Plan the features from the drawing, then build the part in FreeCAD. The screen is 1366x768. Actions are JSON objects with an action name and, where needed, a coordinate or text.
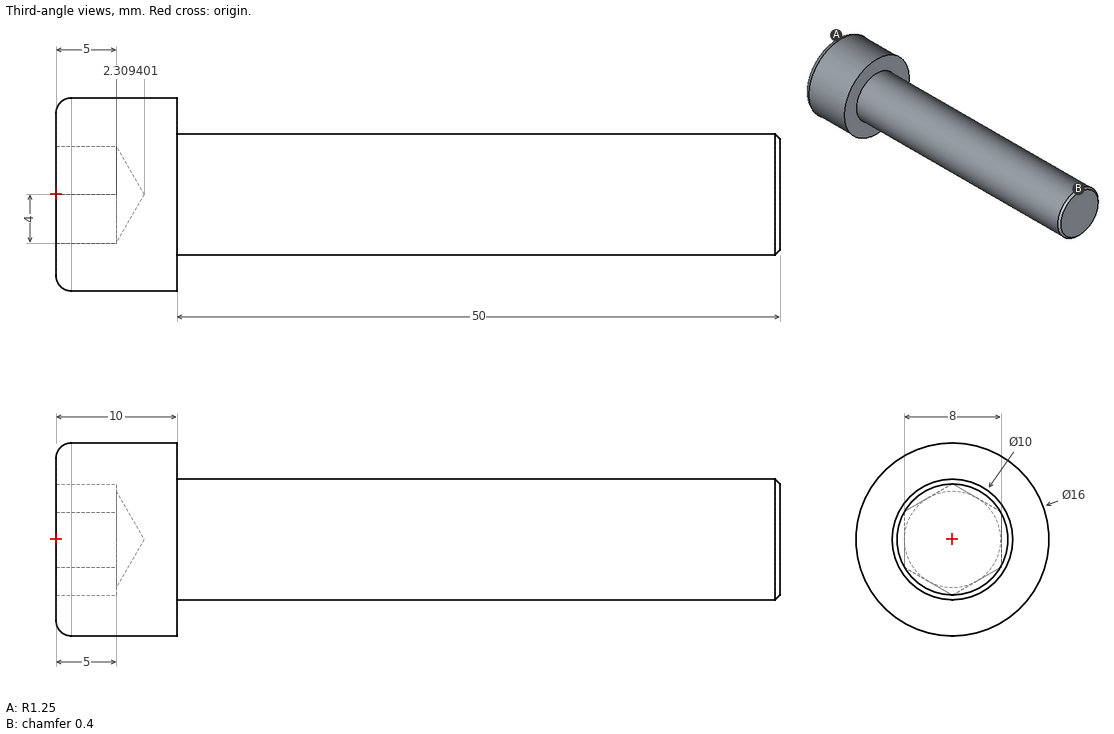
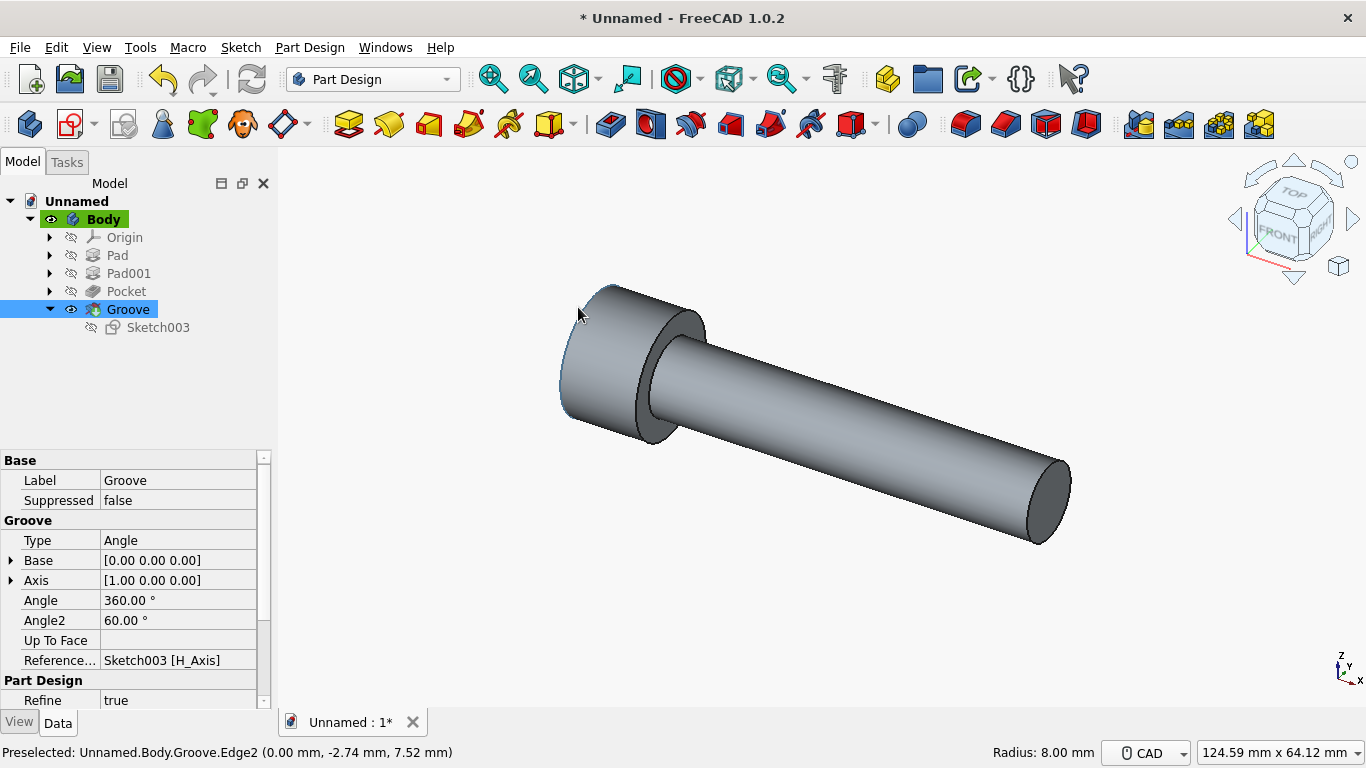
{"action": "left_click", "coordinate": [966, 124]}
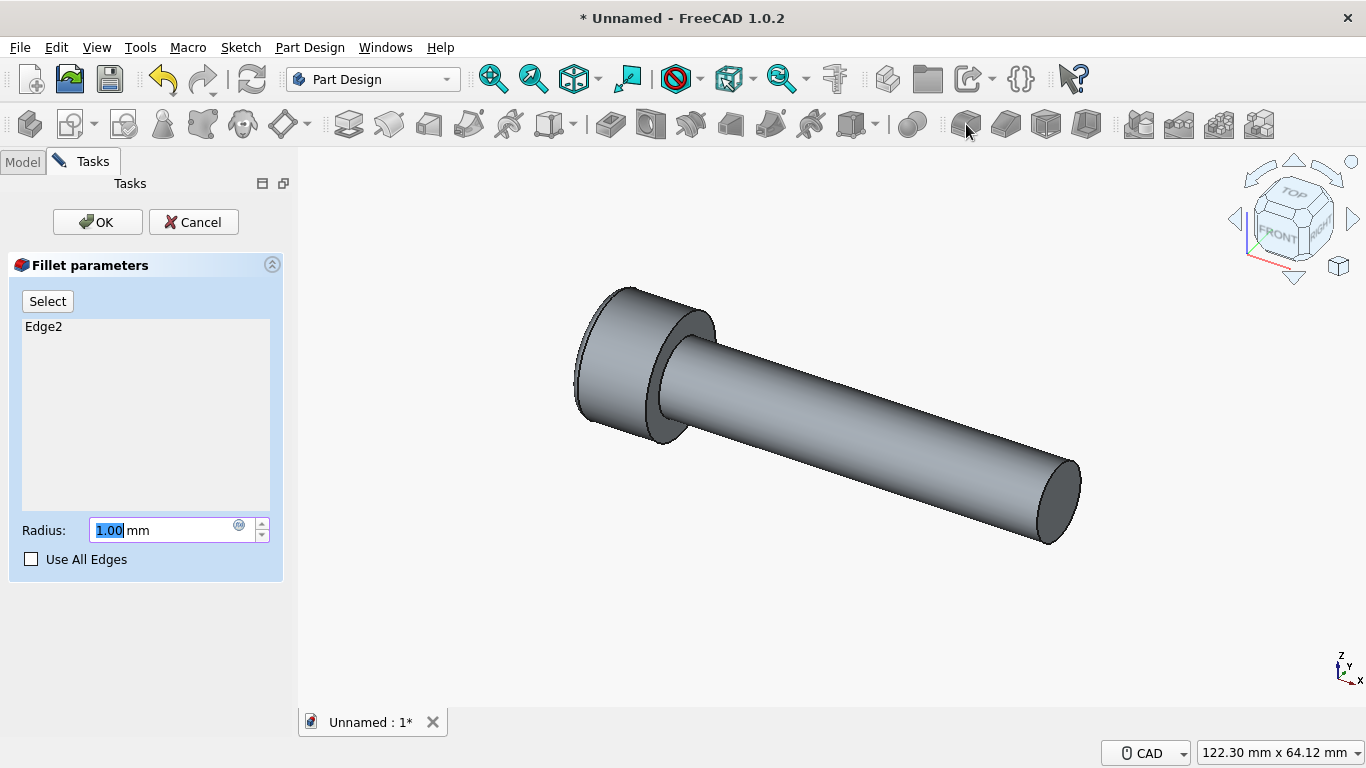
{"action": "type", "text": "1.25"}
{"action": "key", "text": "Tab"}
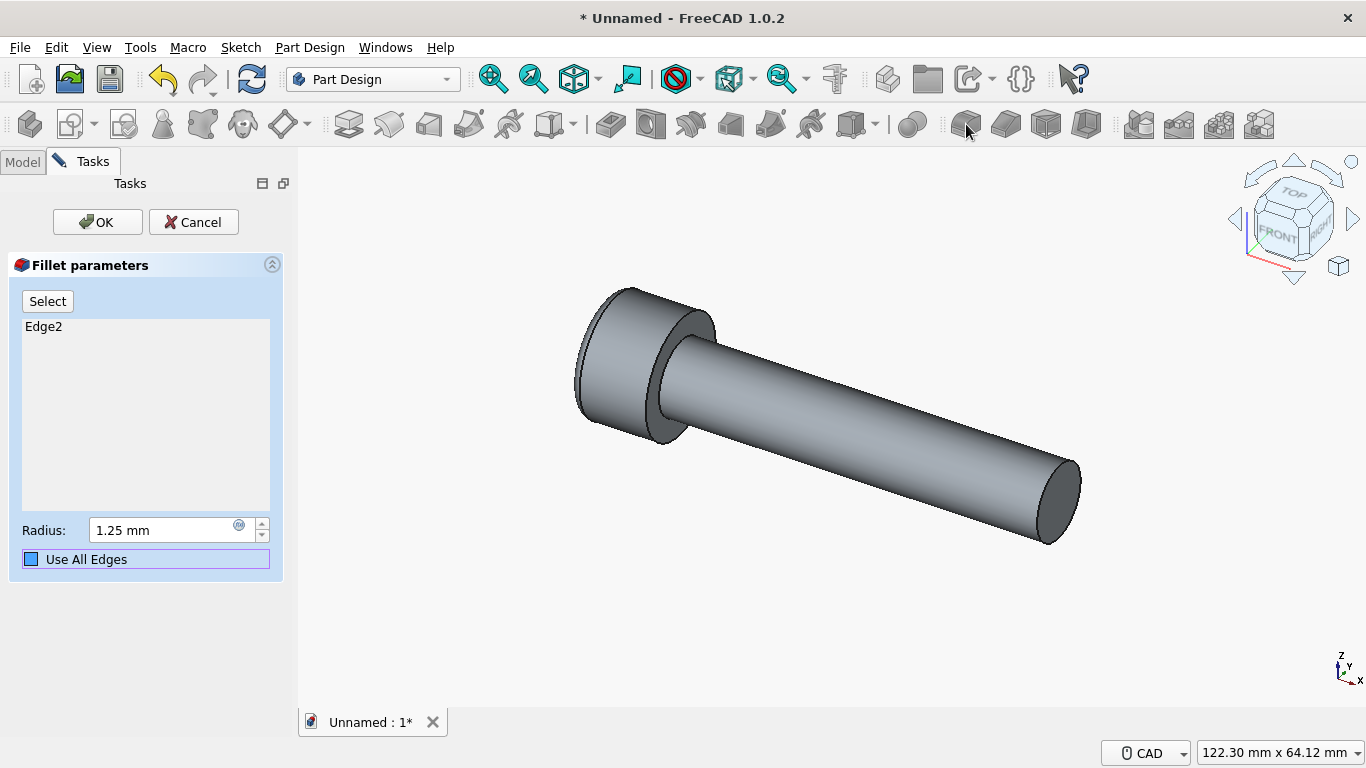
{"action": "left_click", "coordinate": [98, 222]}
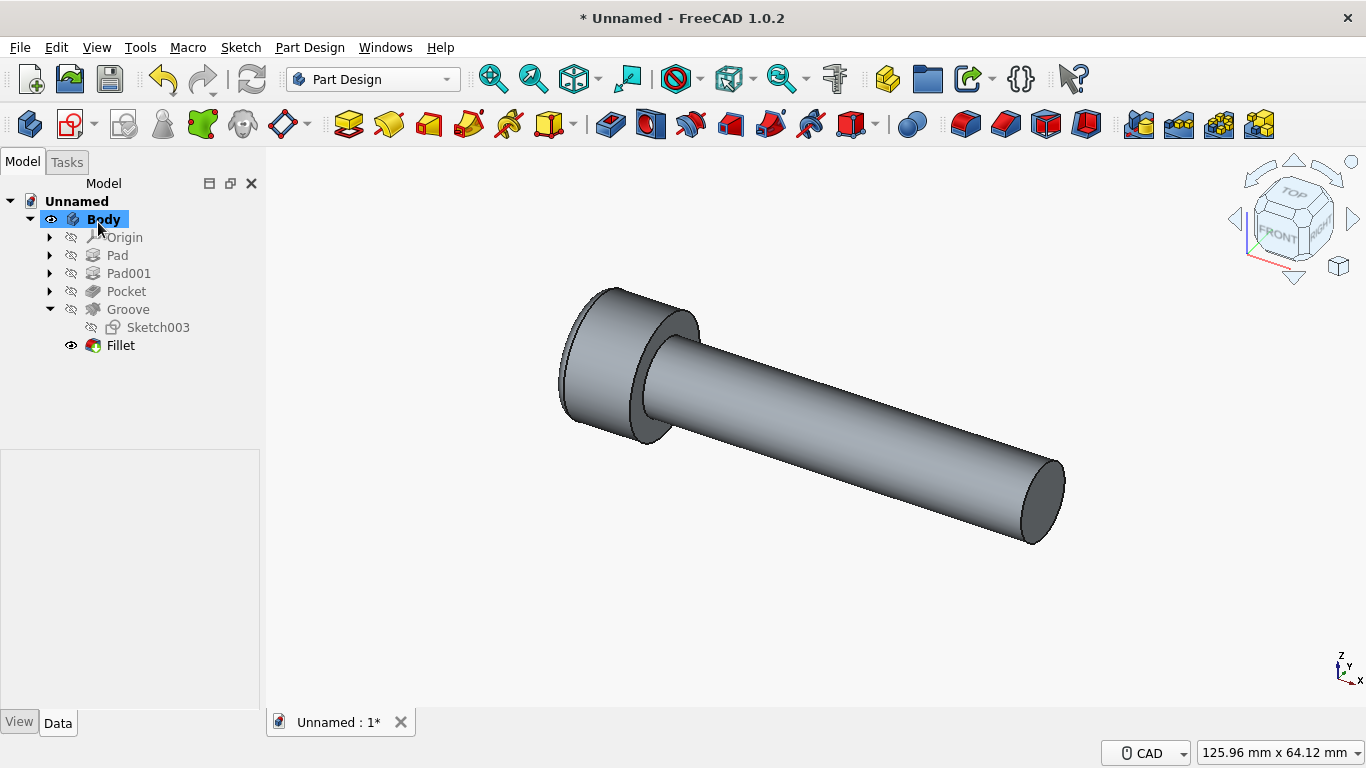
{"action": "left_click", "coordinate": [1021, 523]}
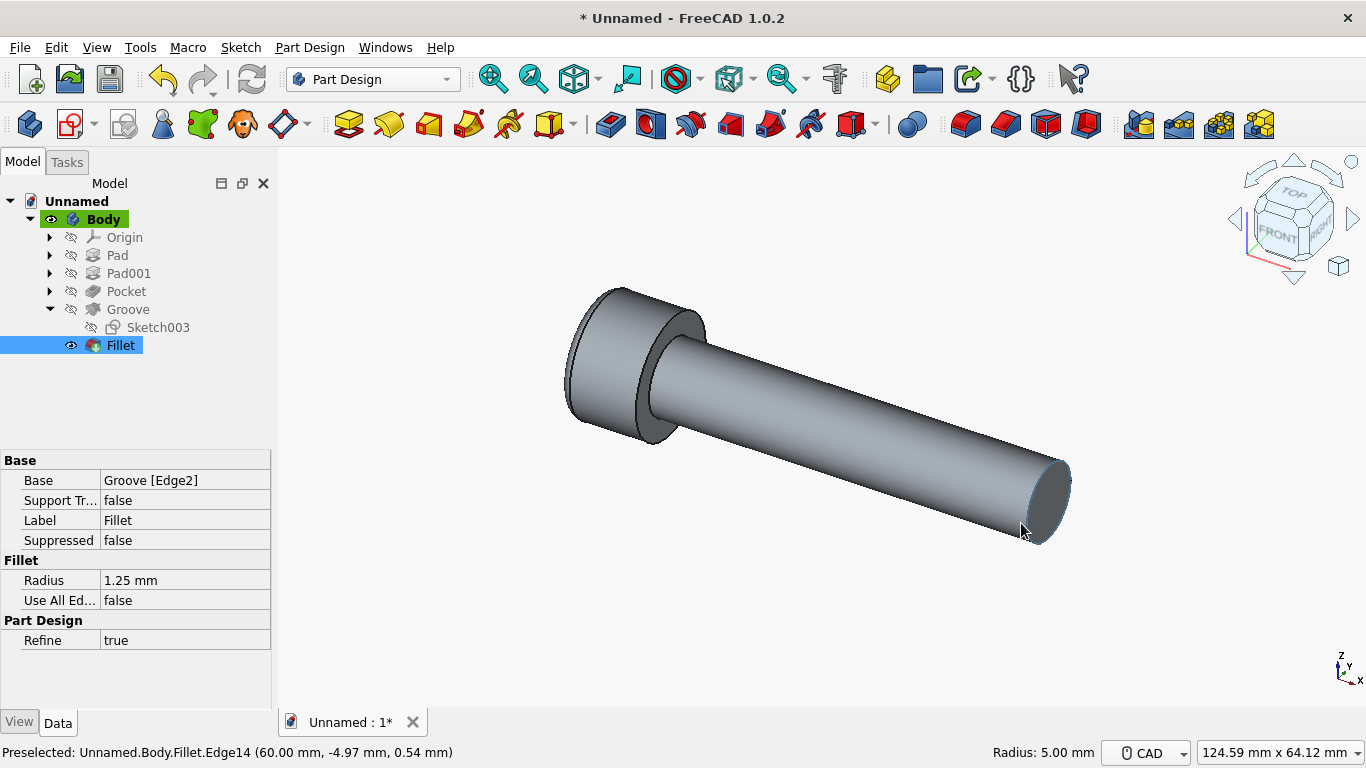
{"action": "left_click", "coordinate": [1006, 124]}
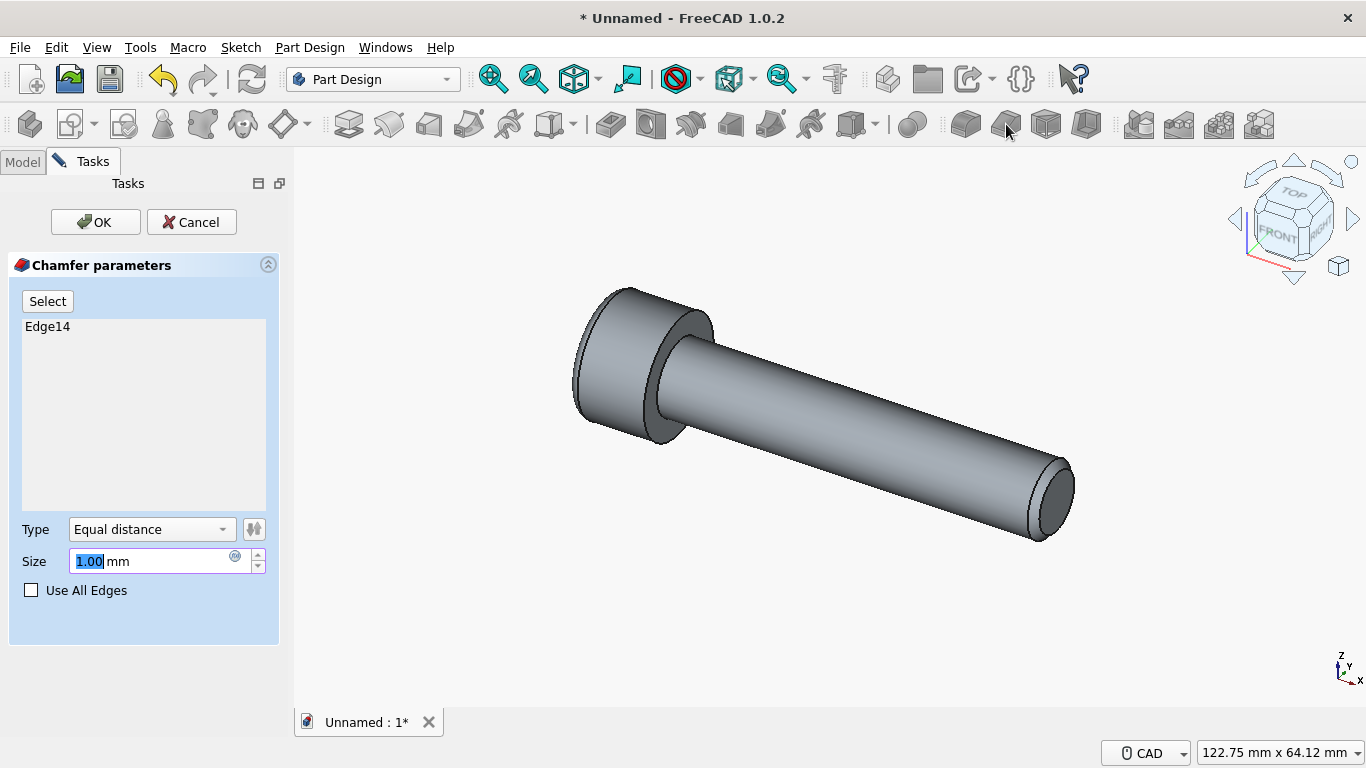
{"action": "type", "text": "0.4"}
{"action": "key", "text": "Tab"}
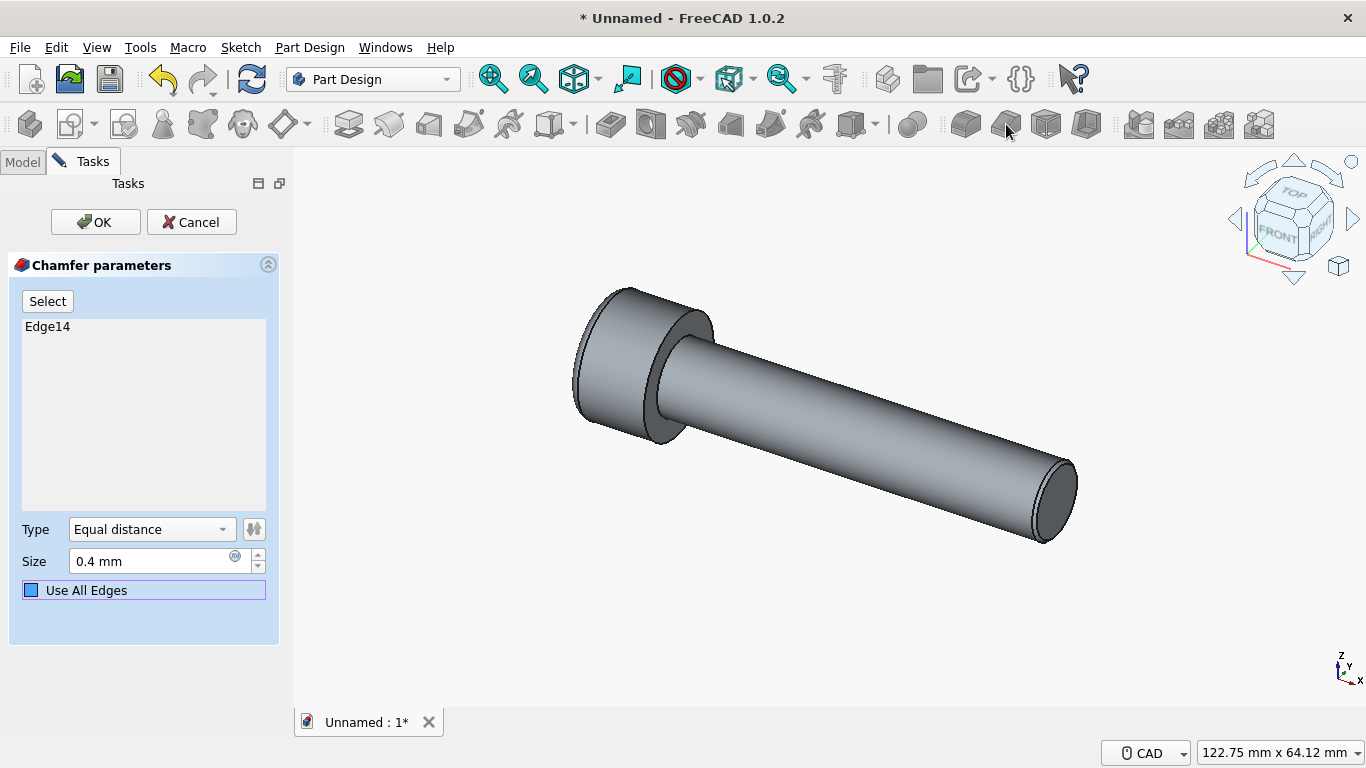
{"action": "left_click", "coordinate": [96, 222]}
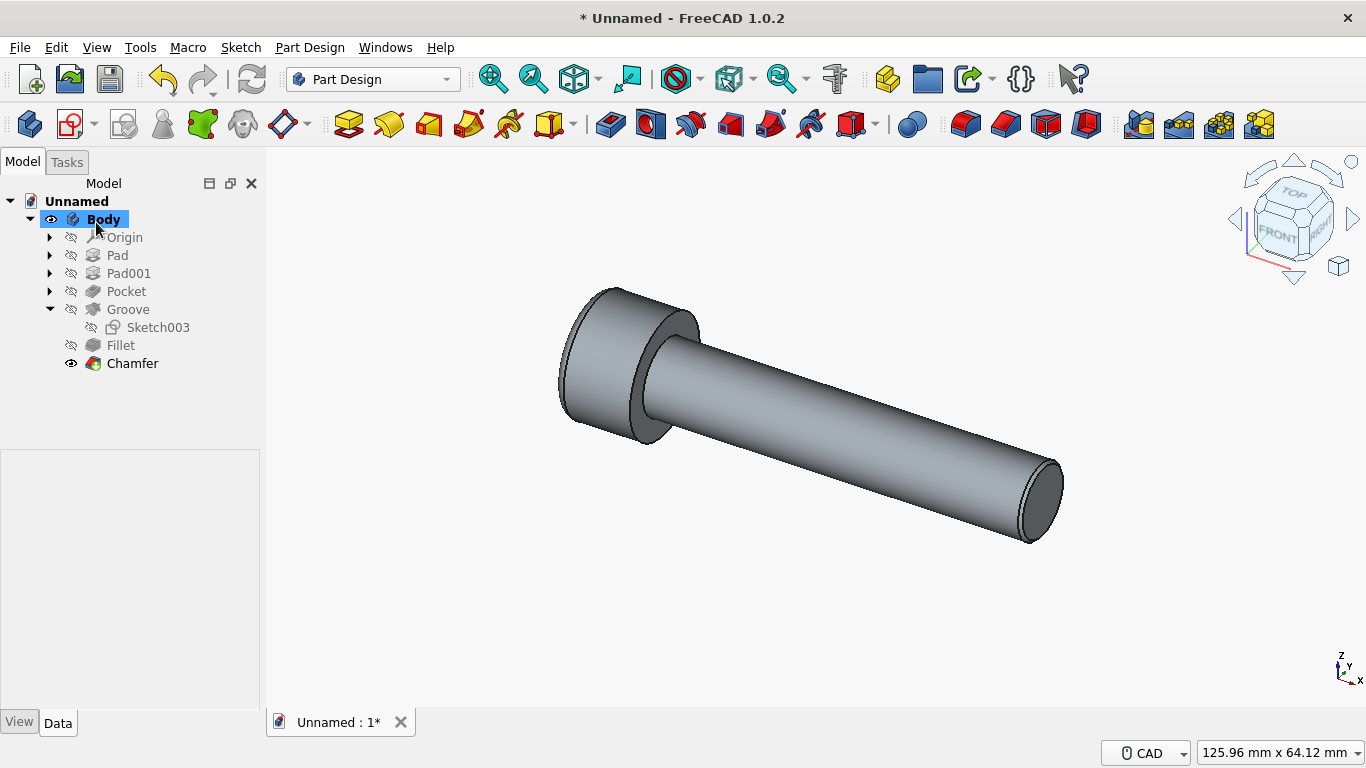
{"action": "key", "text": "0"}